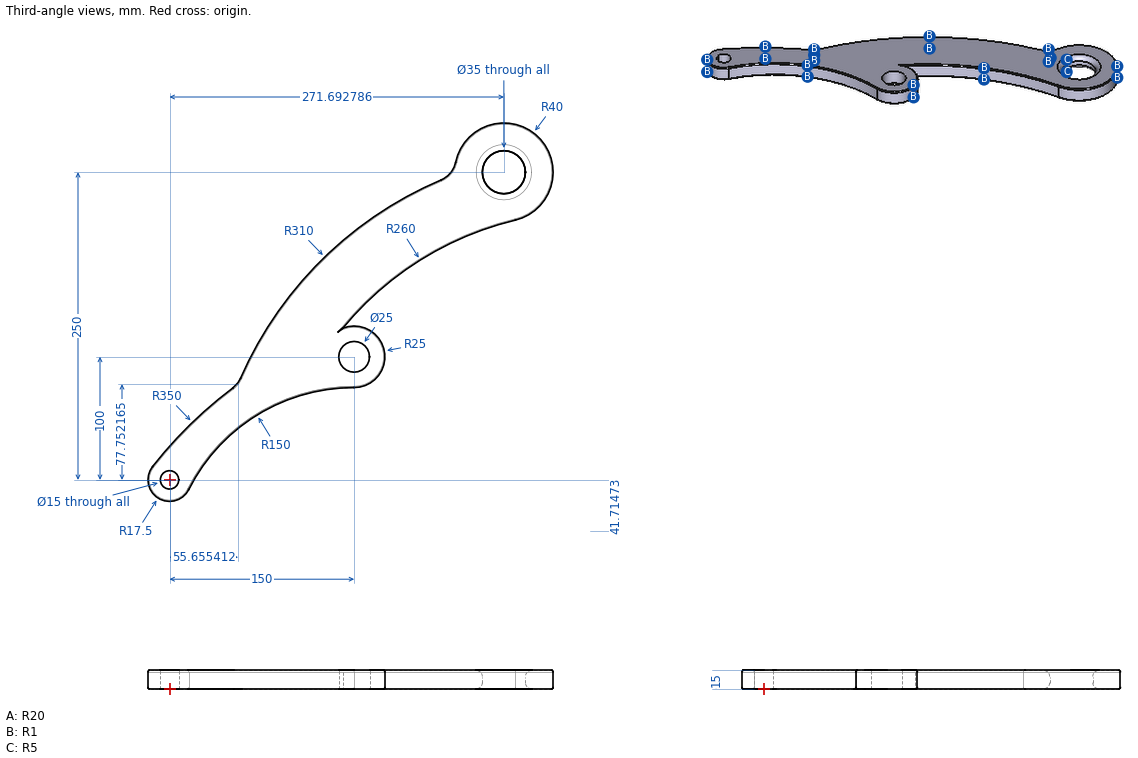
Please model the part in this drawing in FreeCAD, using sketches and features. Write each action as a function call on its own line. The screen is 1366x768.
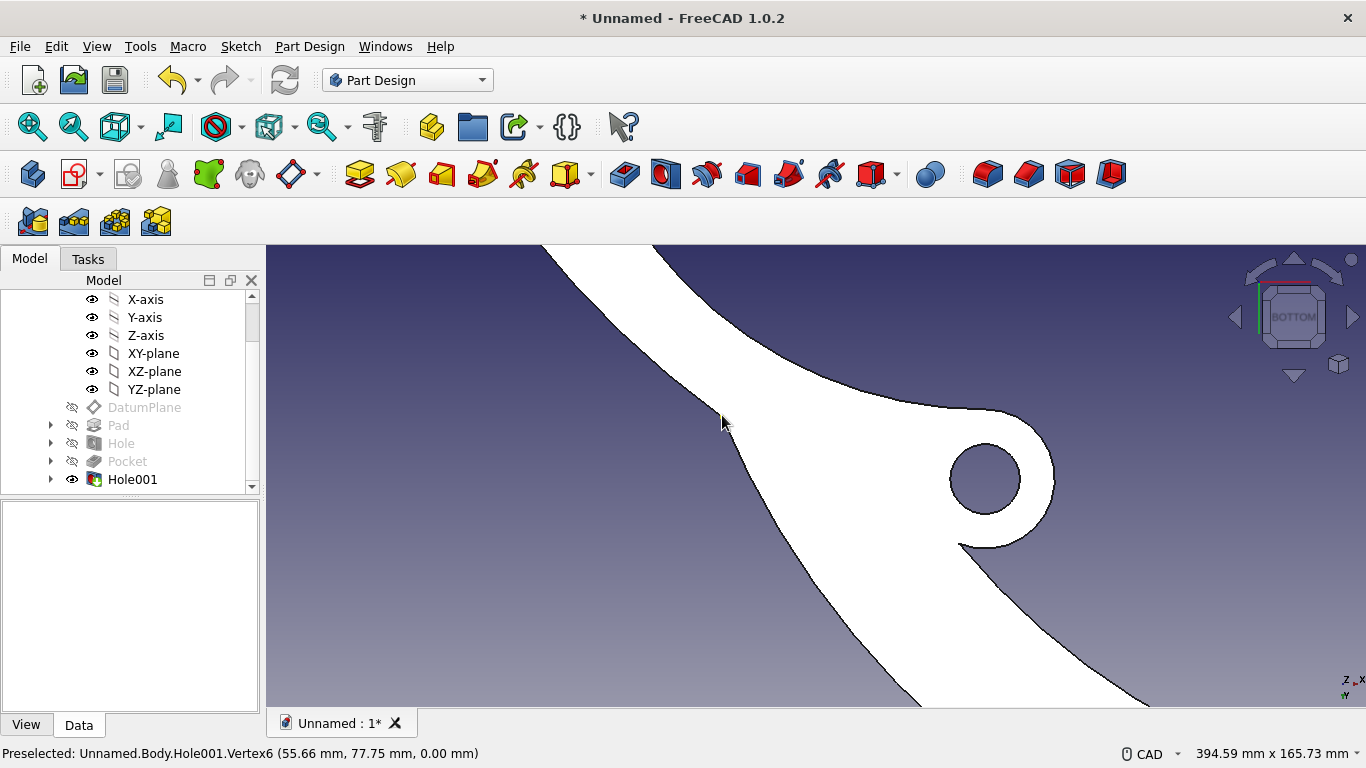
click(33, 128)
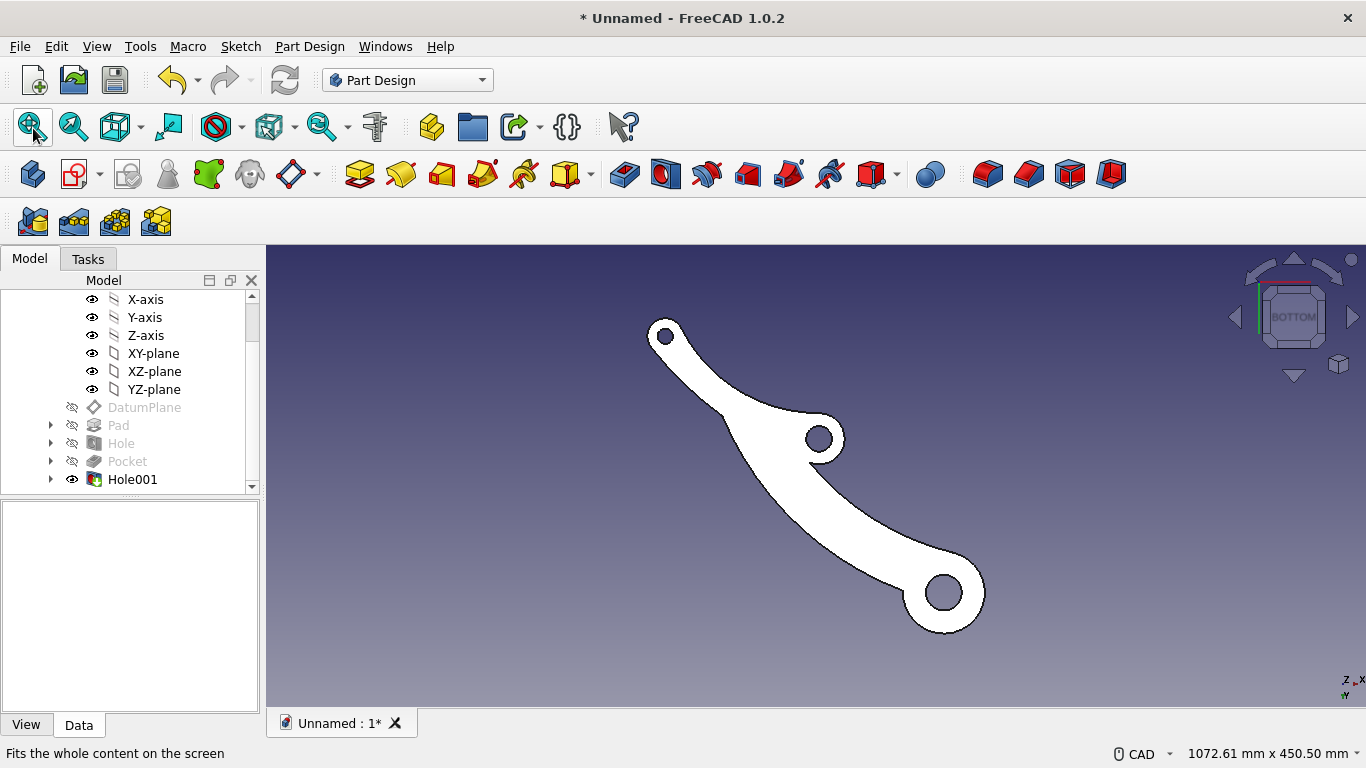
key(4)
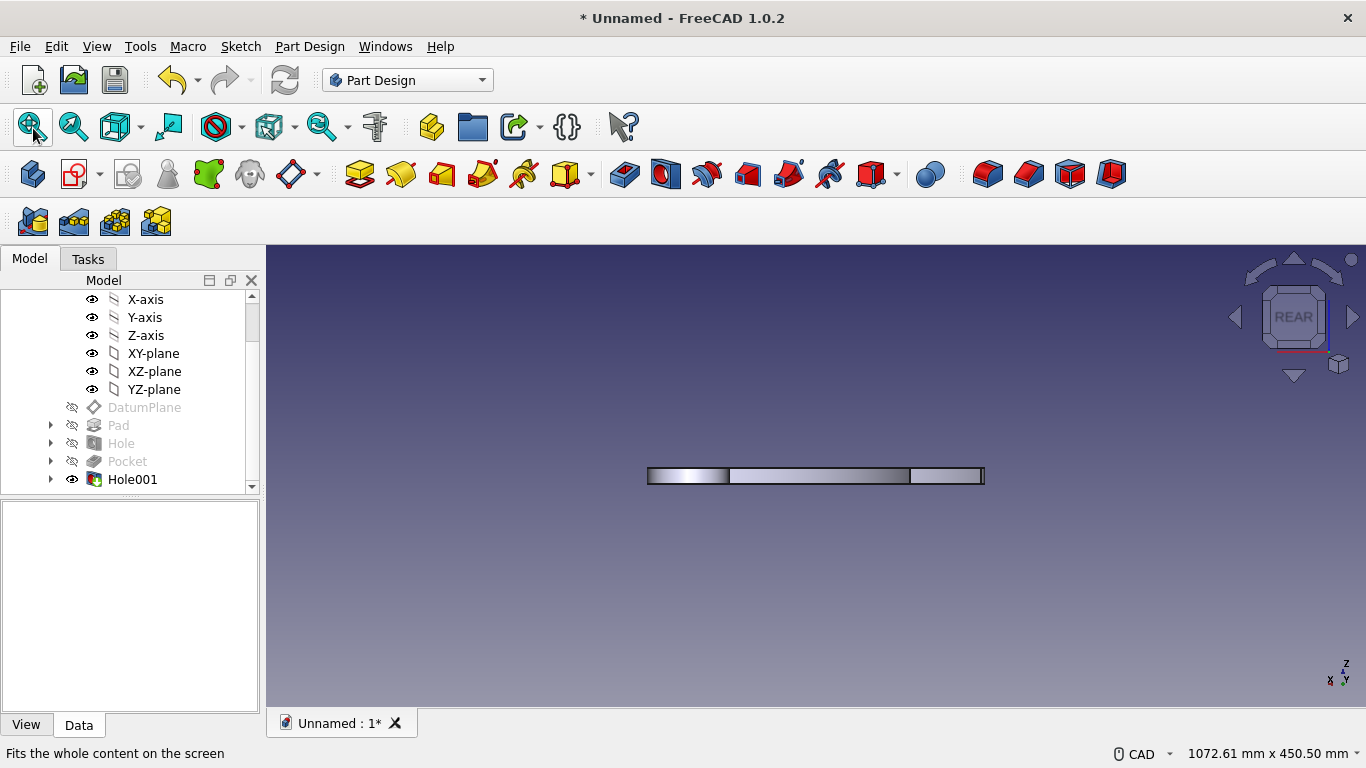
key(v)
key(f)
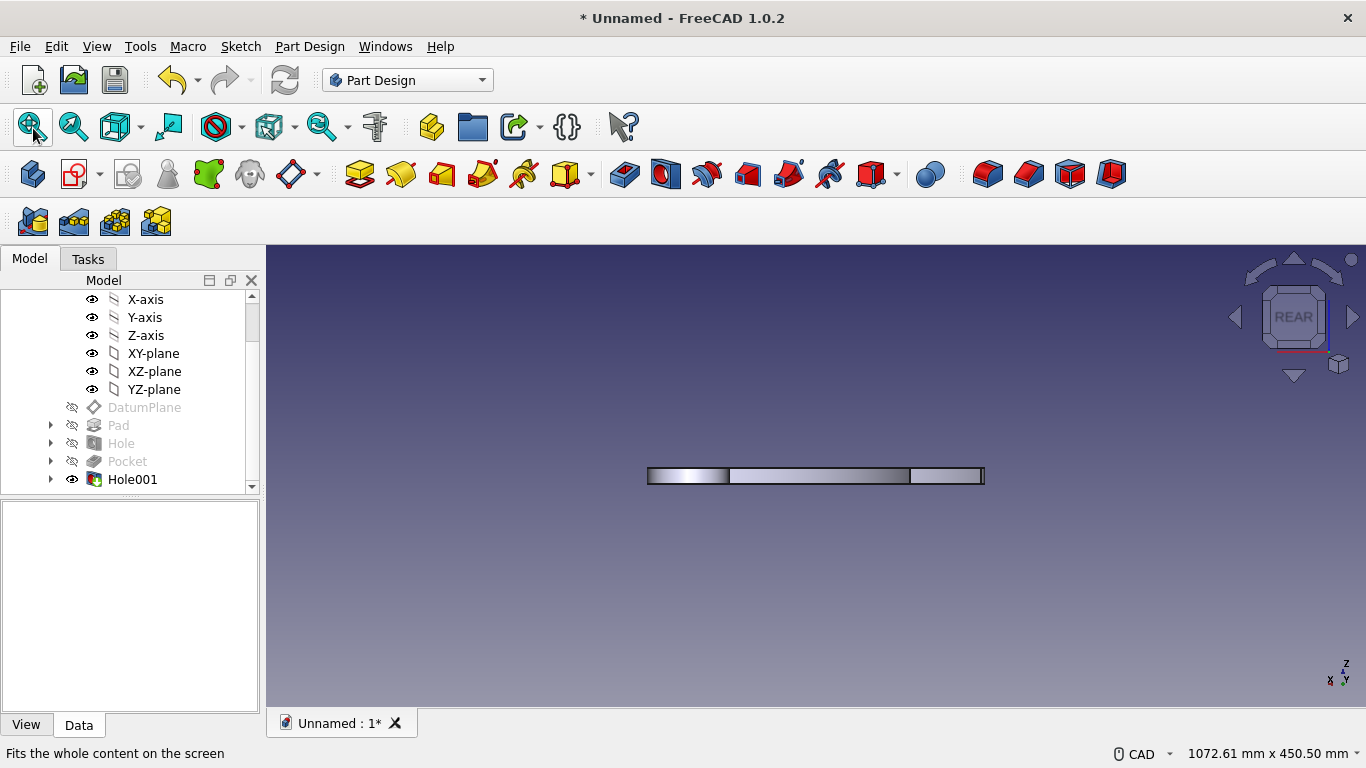
scroll(910, 475, up, 5)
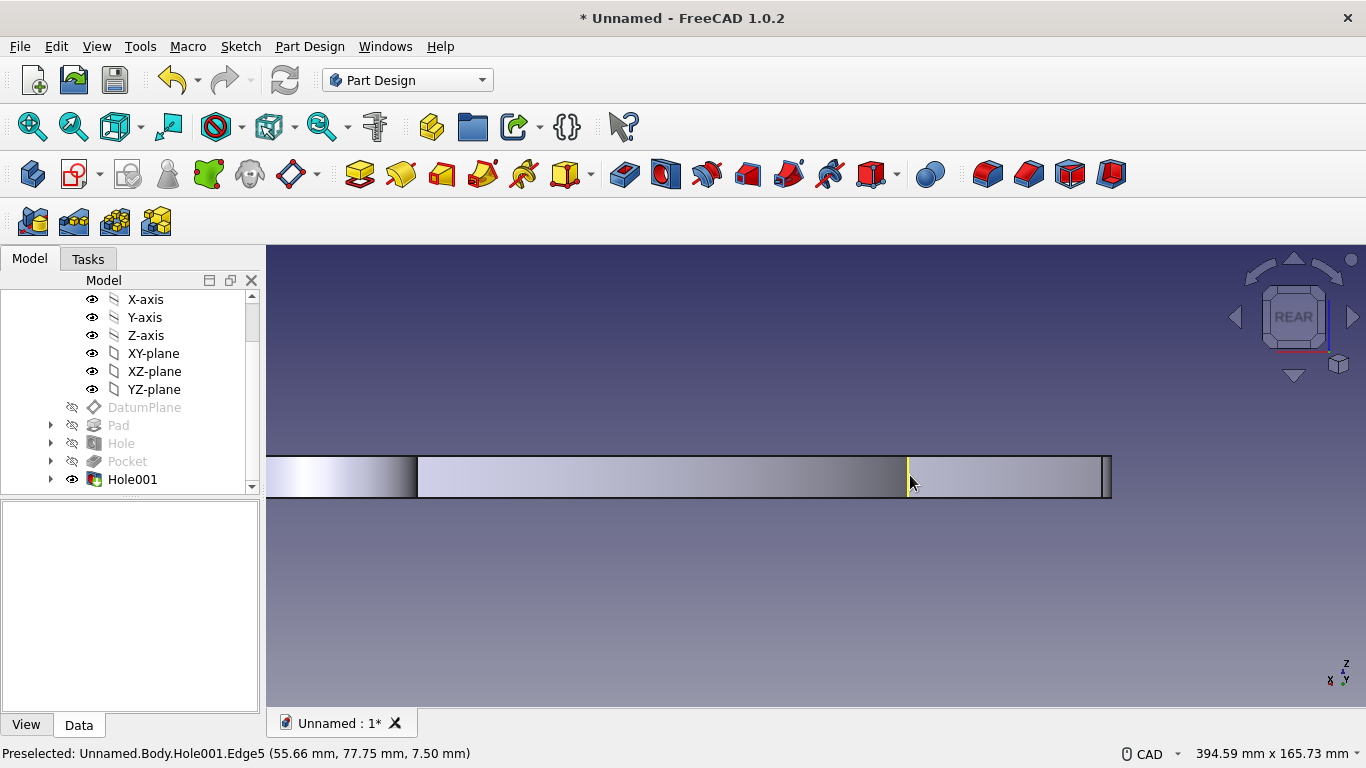
click(33, 128)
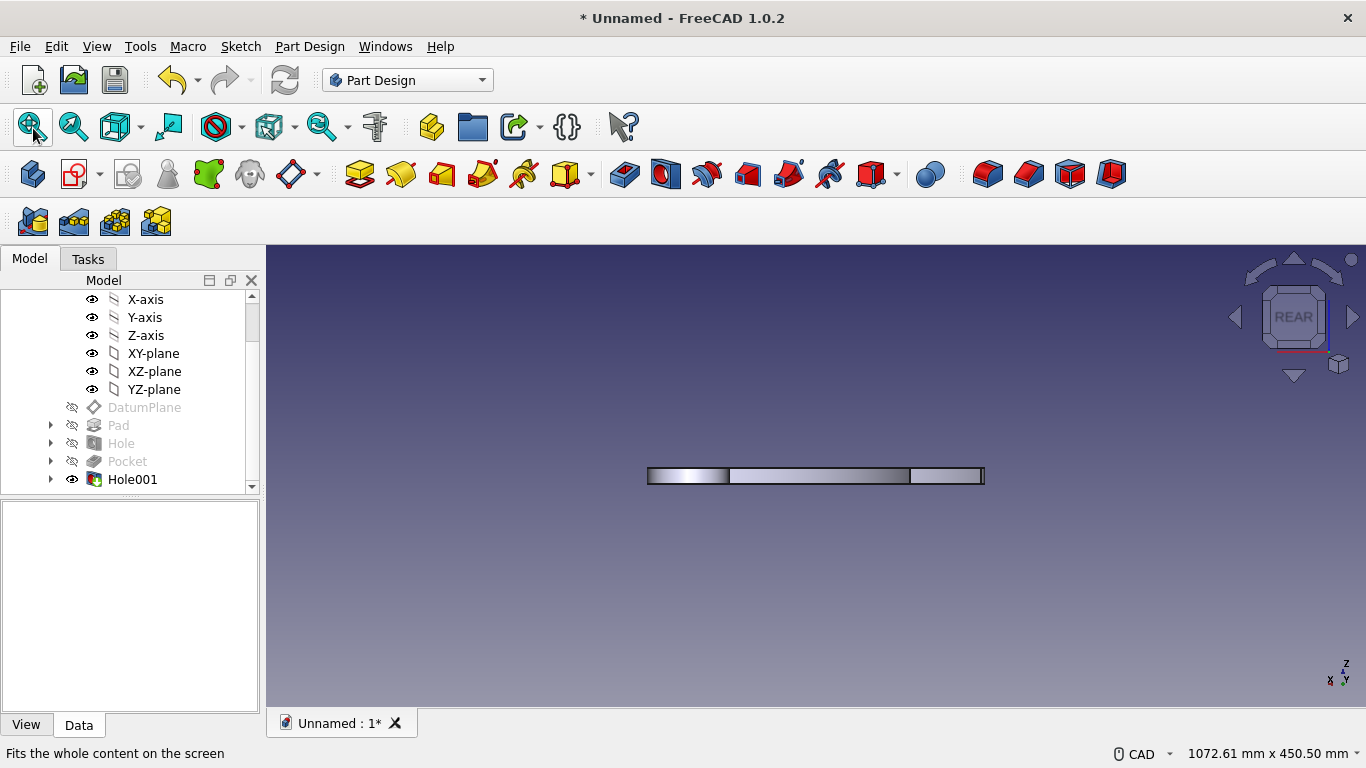
key(6)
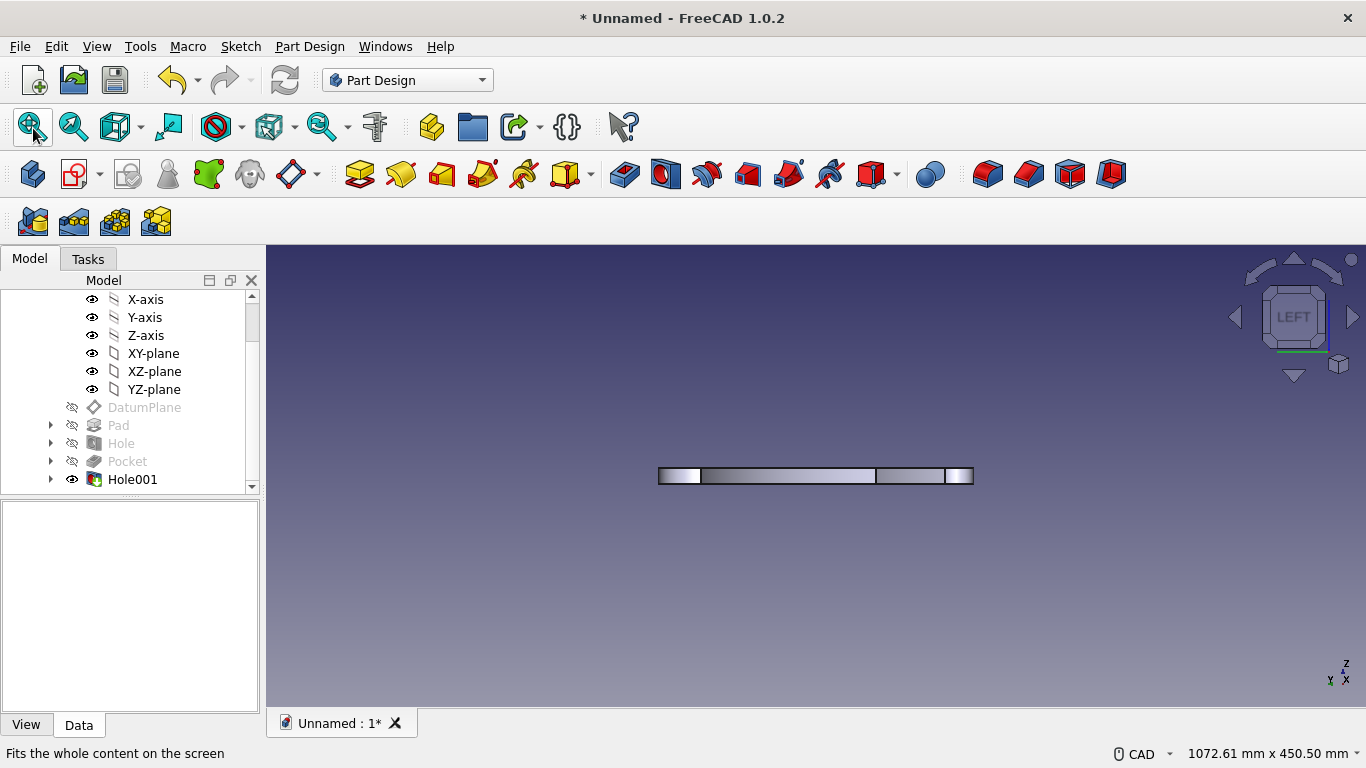
key(v)
key(f)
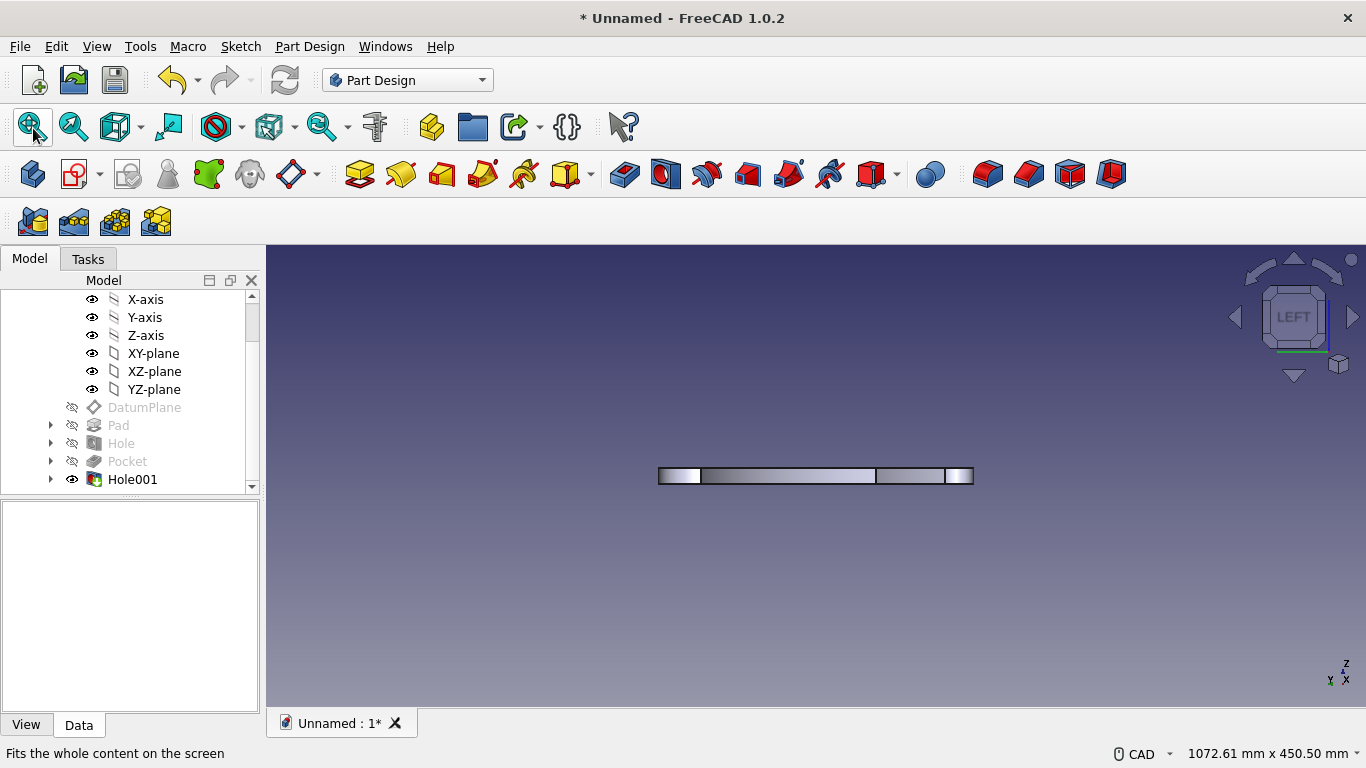
scroll(876, 475, up, 5)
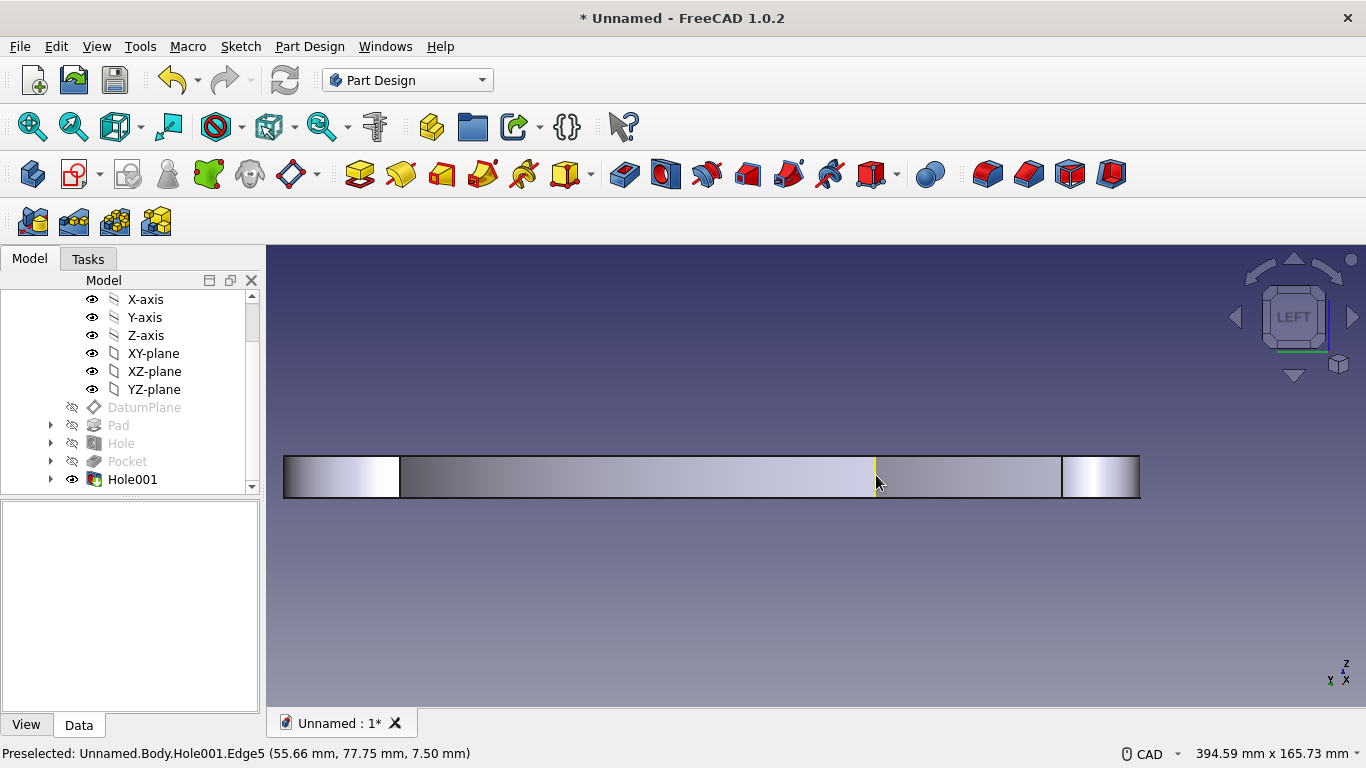
click(33, 128)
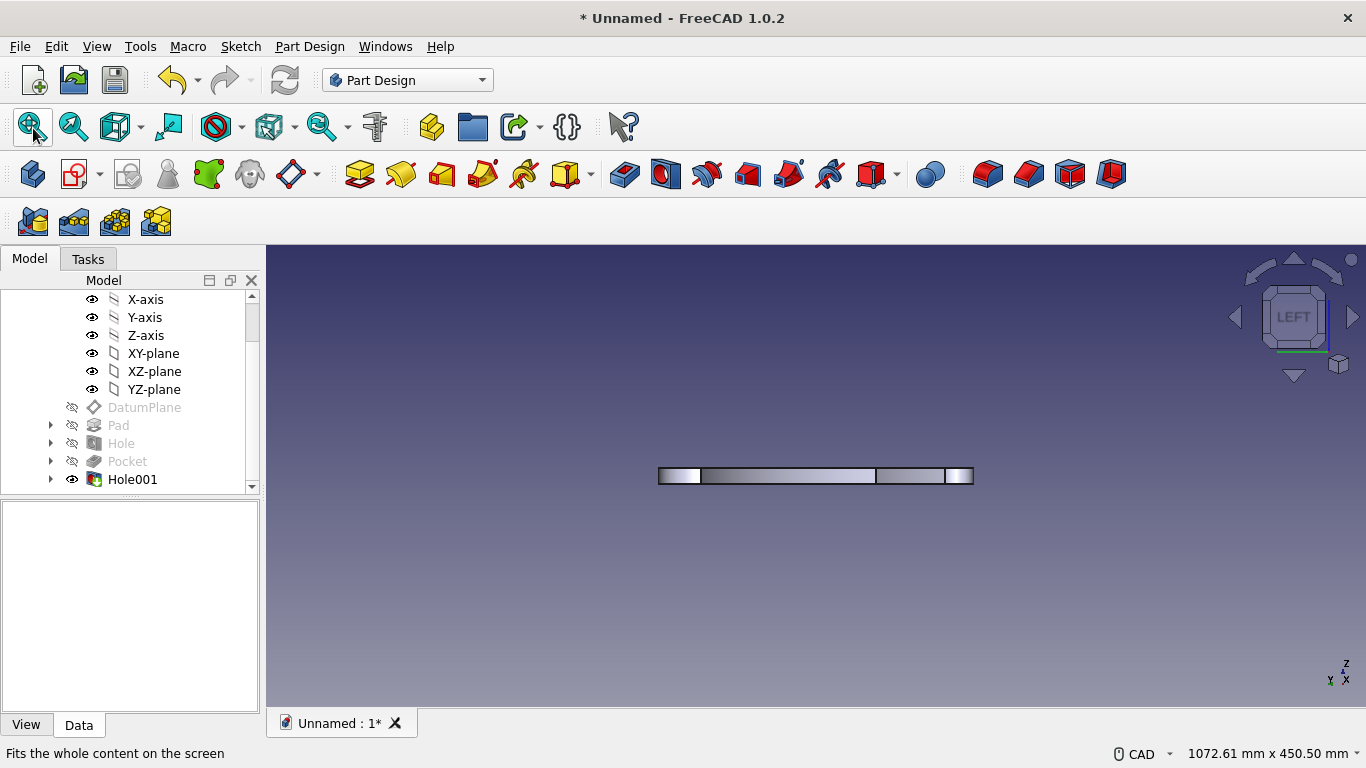
key(v)
key(3)